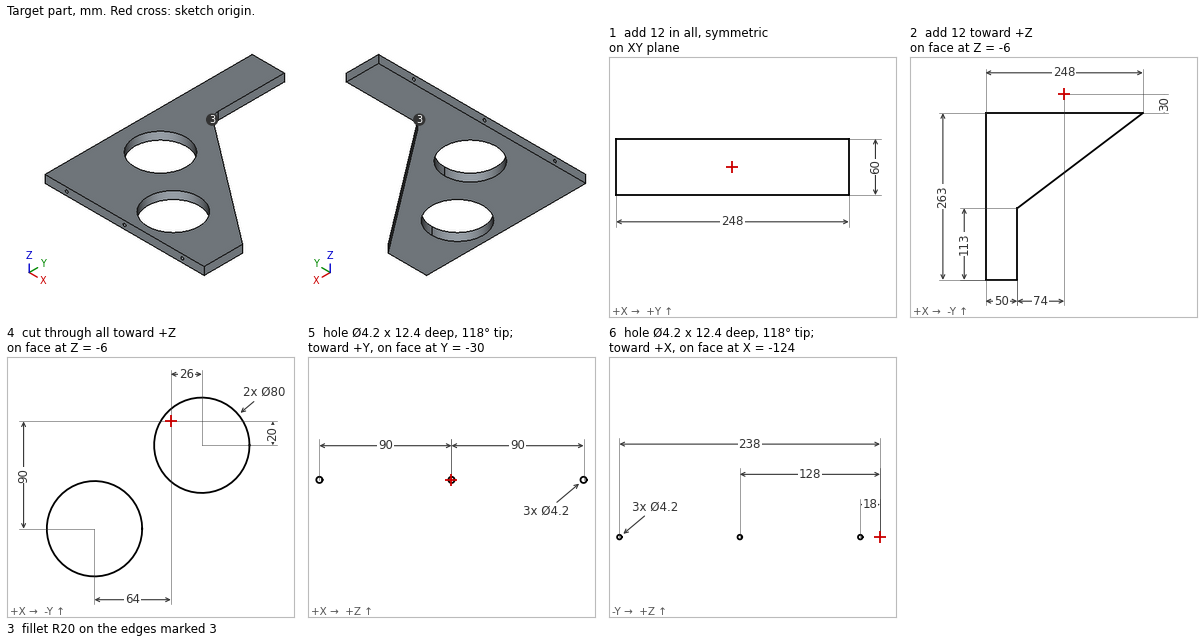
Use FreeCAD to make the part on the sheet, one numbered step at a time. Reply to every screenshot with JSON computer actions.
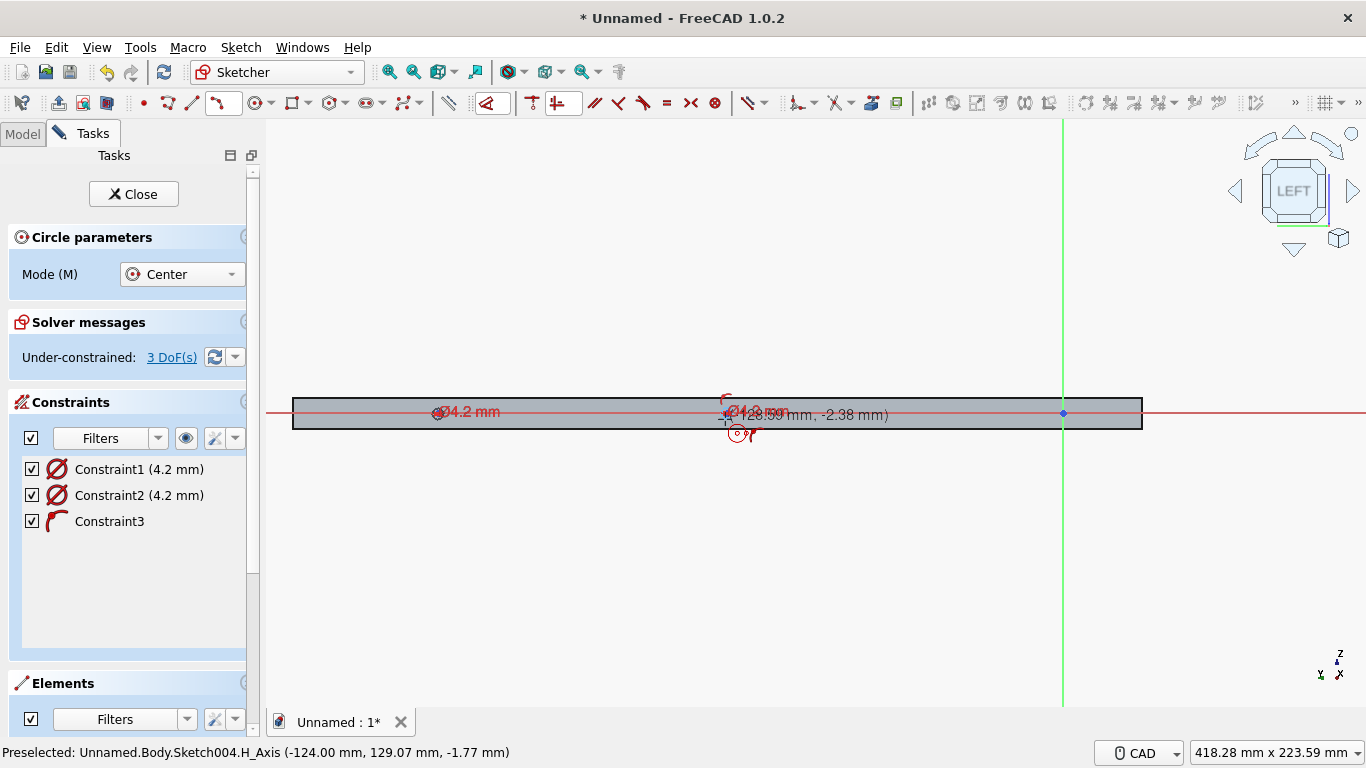
{"action": "scroll", "coordinate": [1016, 413], "scroll_direction": "up", "scroll_amount": 8}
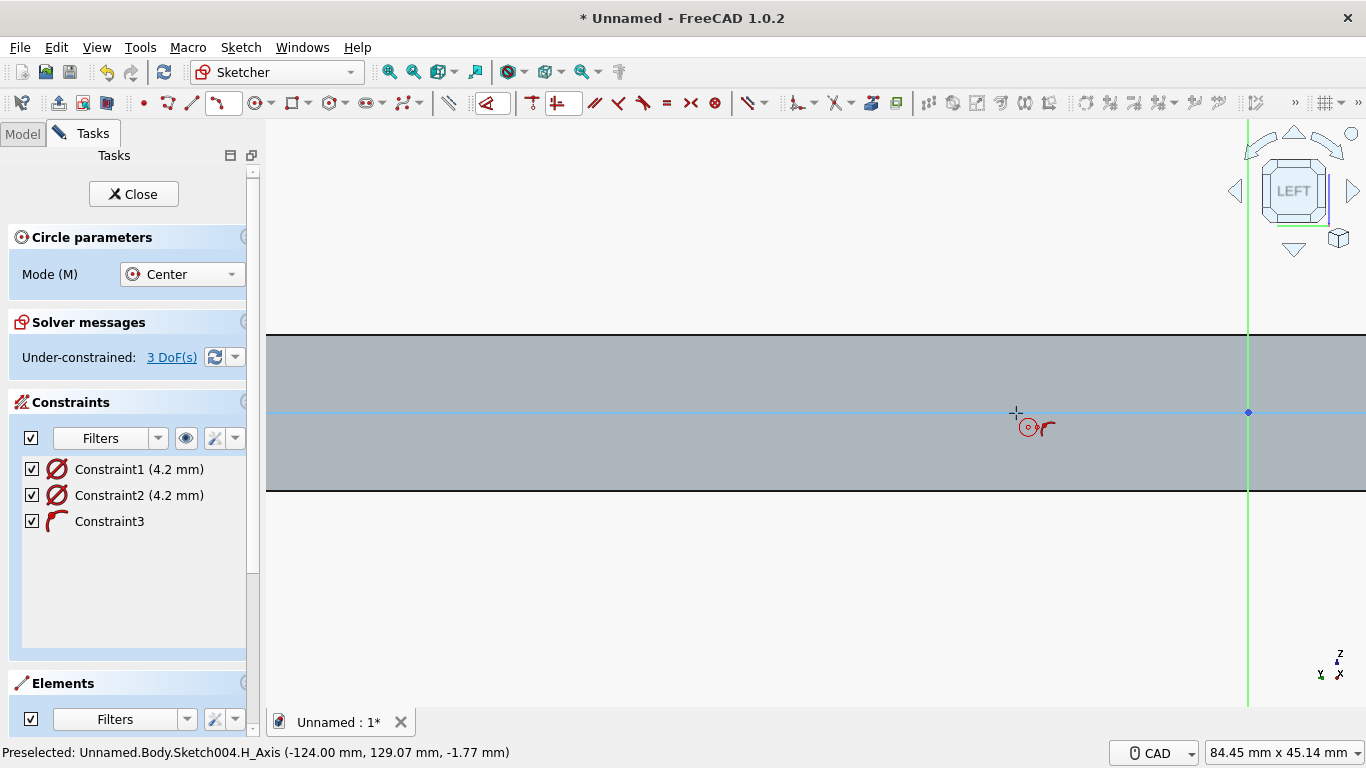
{"action": "scroll", "coordinate": [1016, 413], "scroll_direction": "down", "scroll_amount": 8}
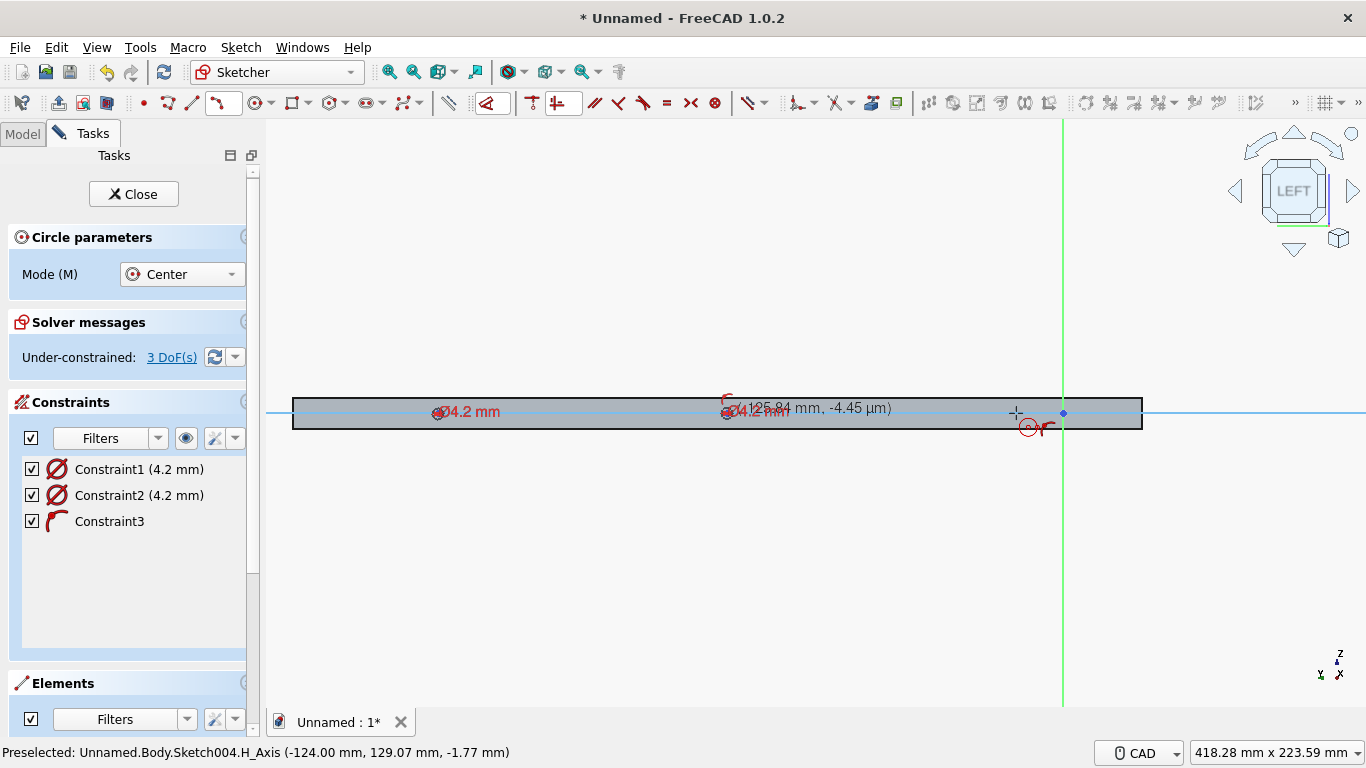
{"action": "left_click", "coordinate": [1016, 413]}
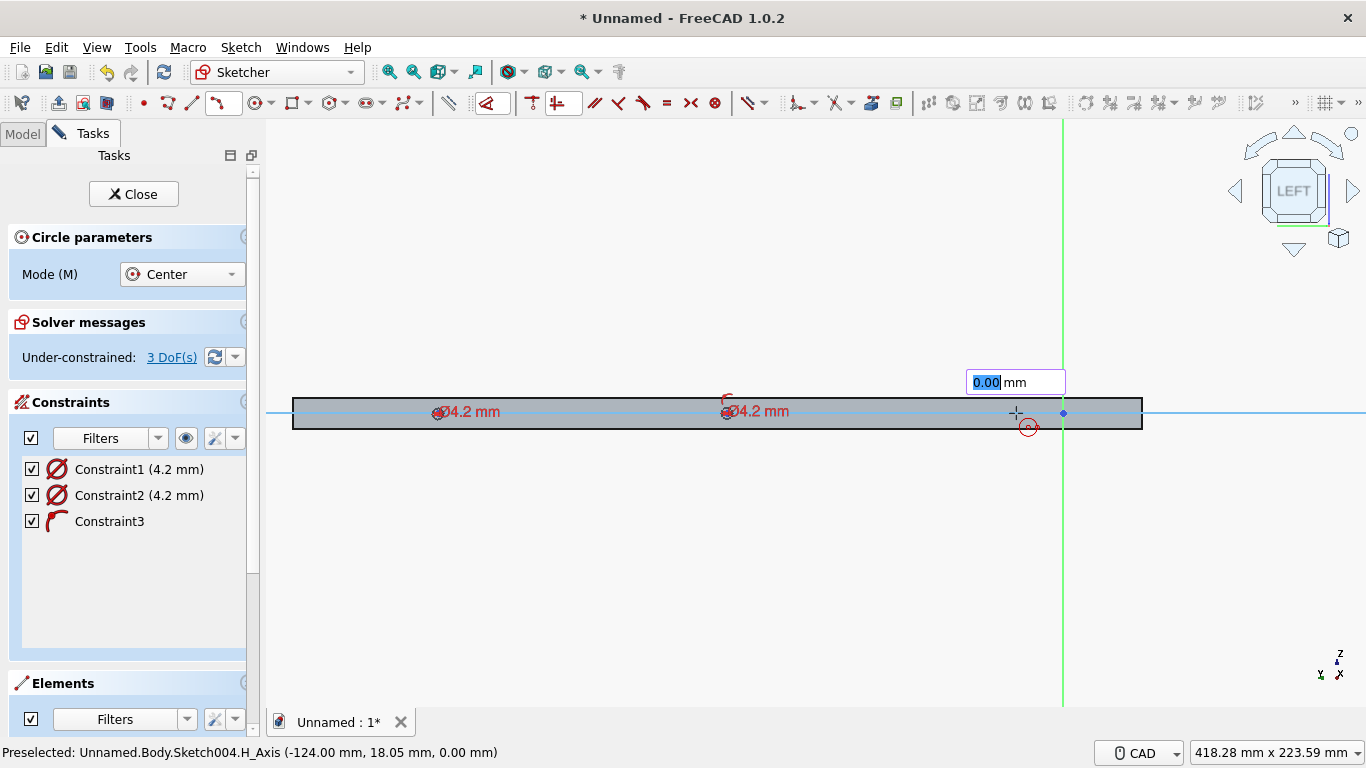
{"action": "scroll", "coordinate": [1014, 419], "scroll_direction": "up", "scroll_amount": 6}
{"action": "mouse_move", "coordinate": [1013, 416]}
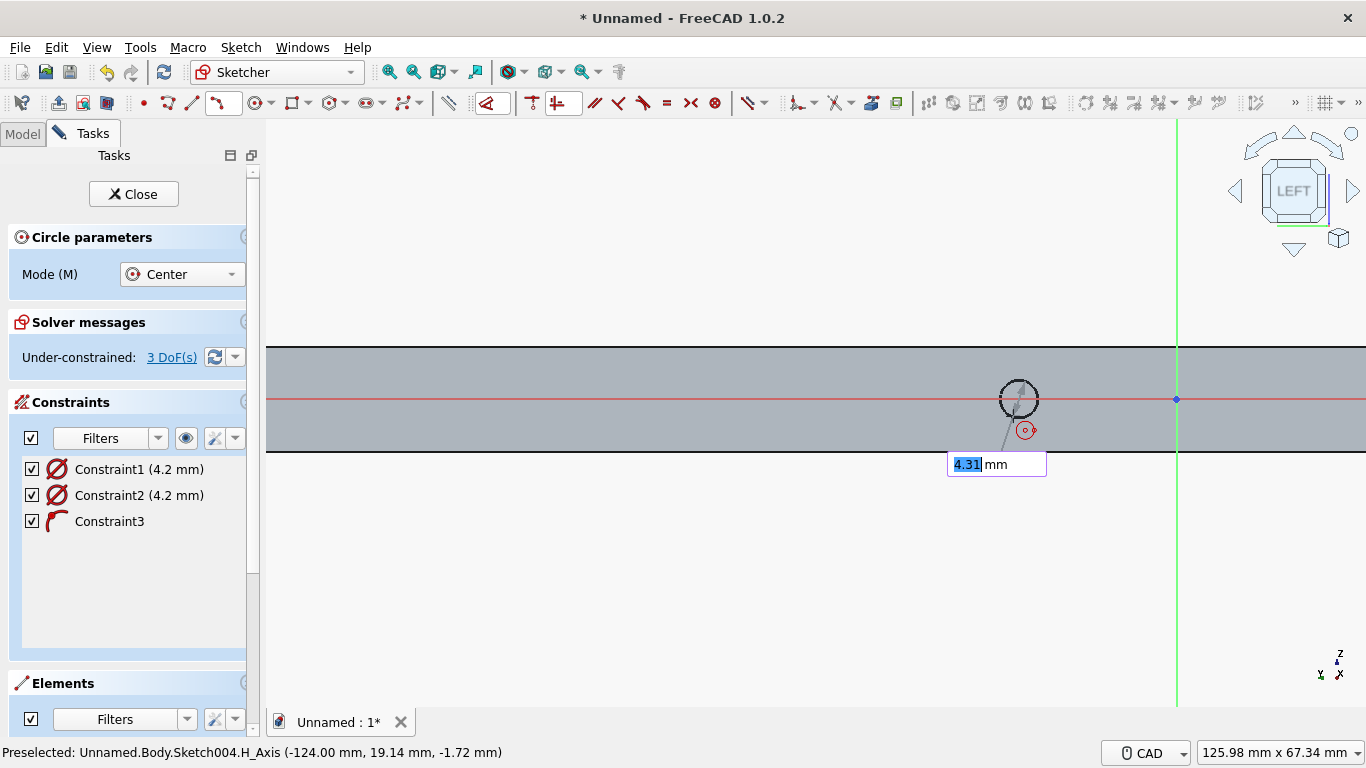
{"action": "type", "text": "4.2"}
{"action": "key", "text": "Return"}
{"action": "key", "text": "Escape"}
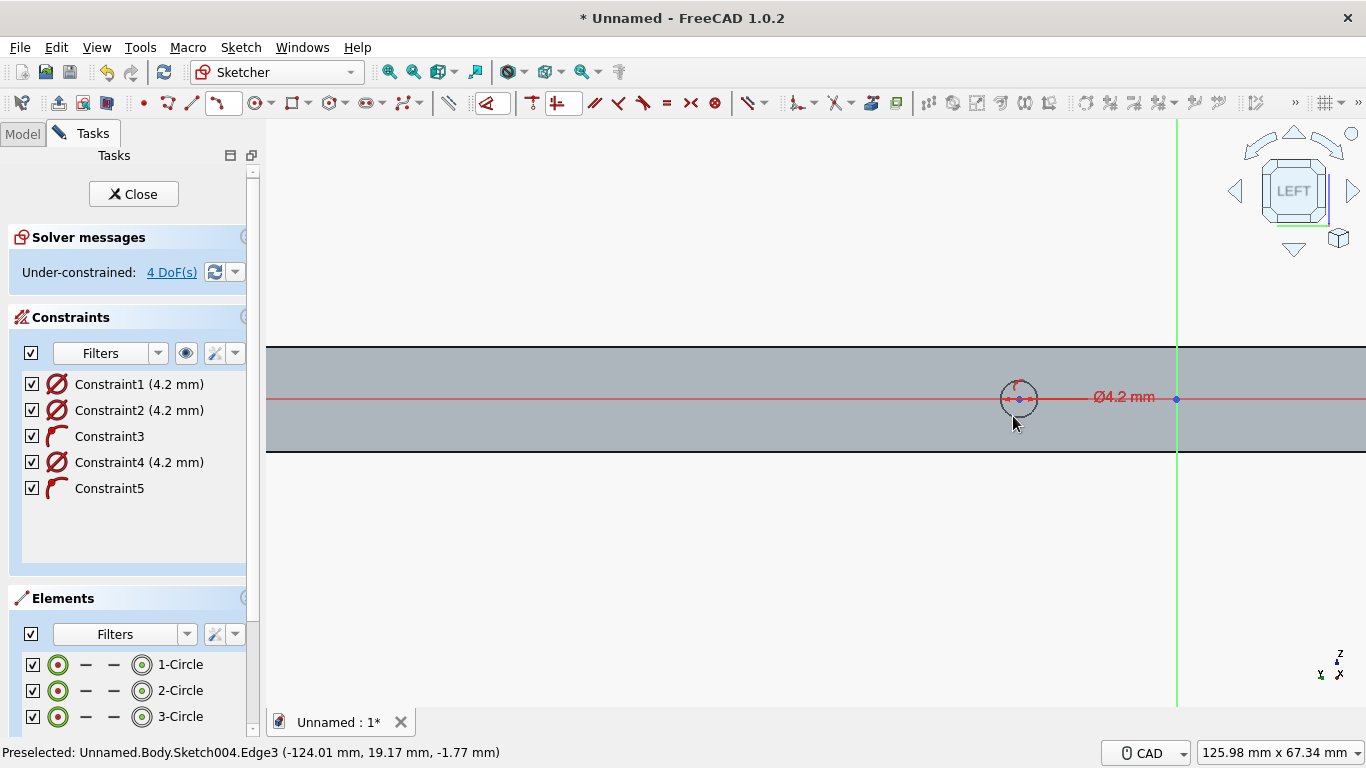
{"action": "scroll", "coordinate": [1014, 419], "scroll_direction": "down", "scroll_amount": 6}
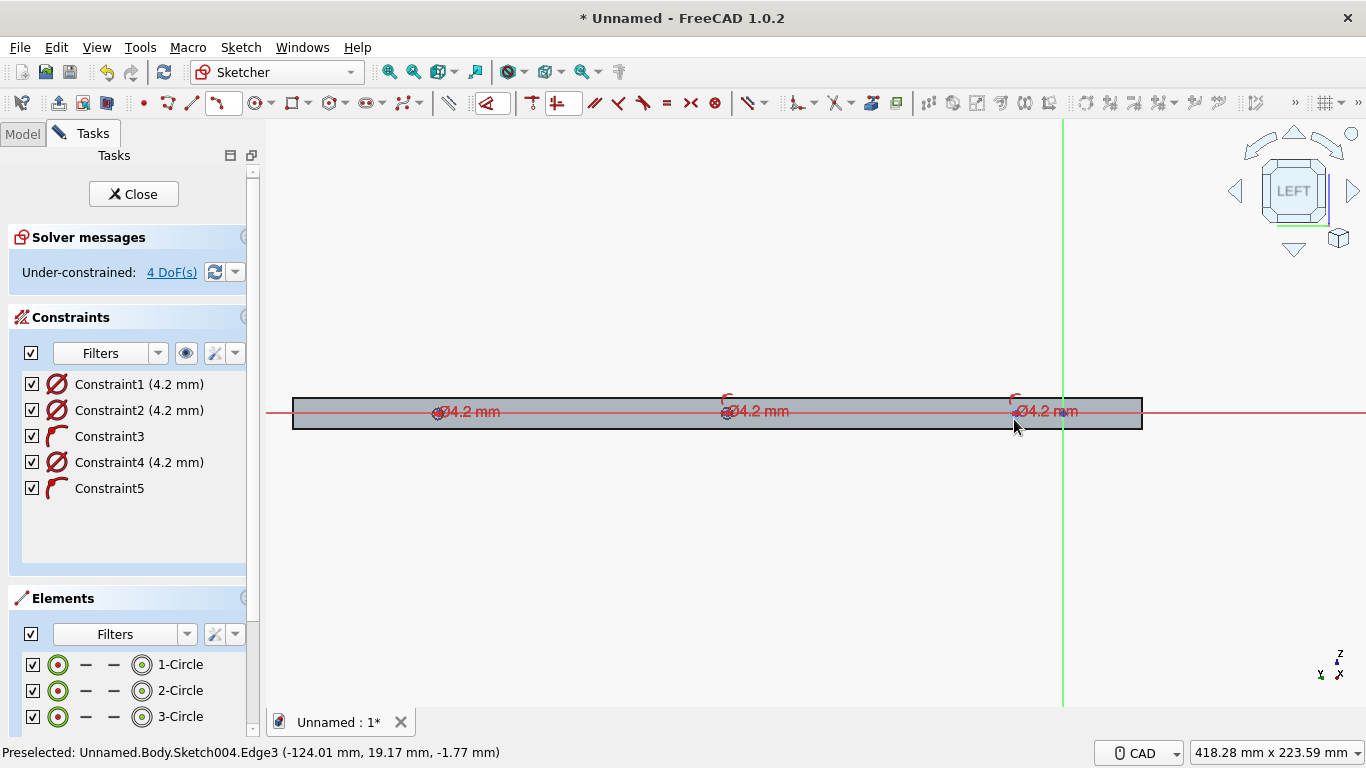
{"action": "left_click", "coordinate": [438, 414]}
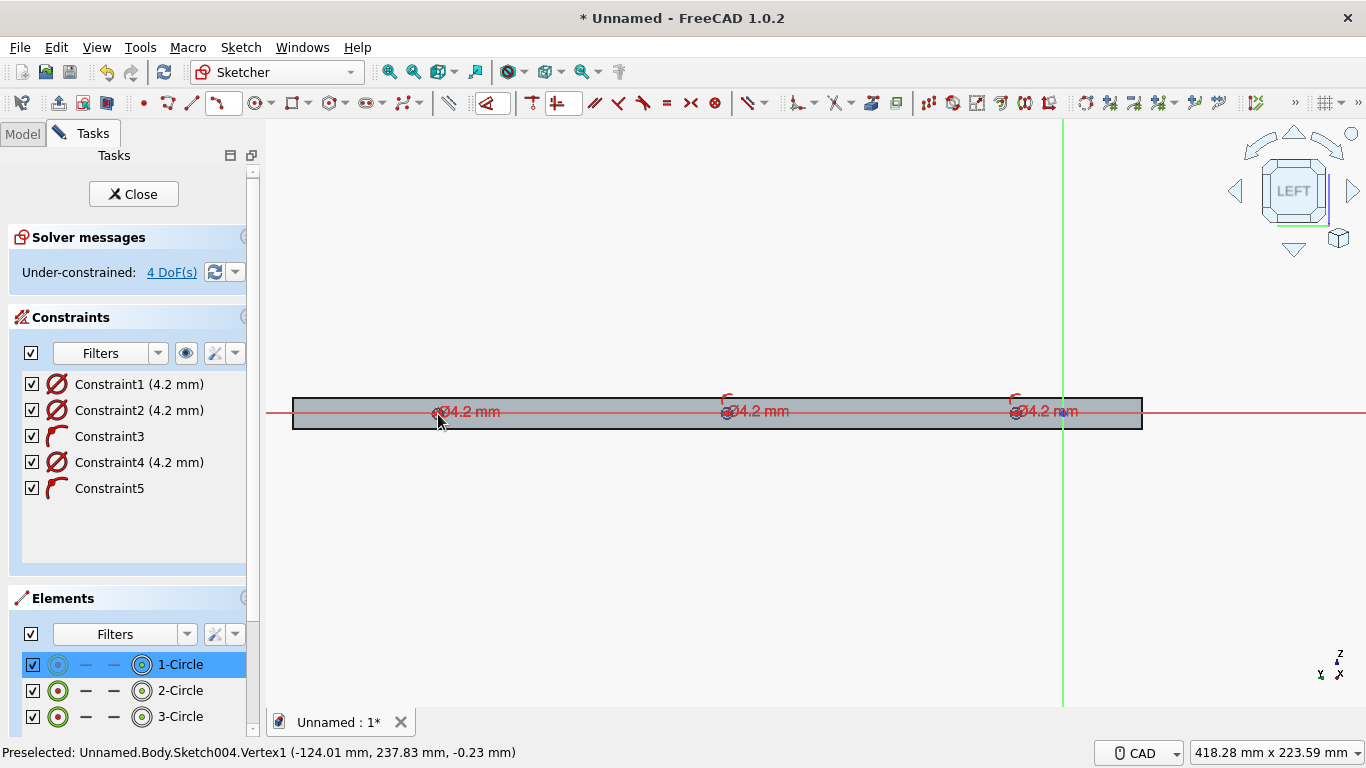
{"action": "left_click", "coordinate": [359, 413]}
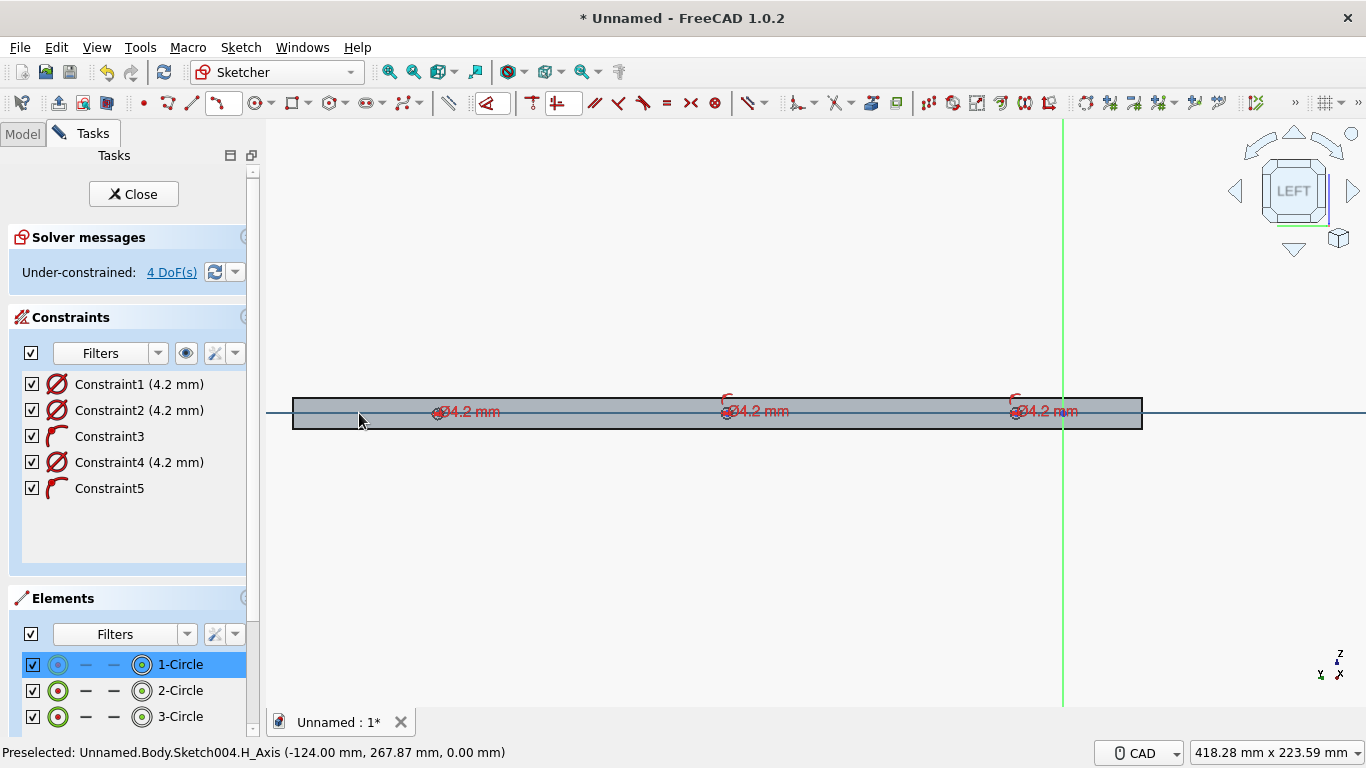
{"action": "key", "text": "c"}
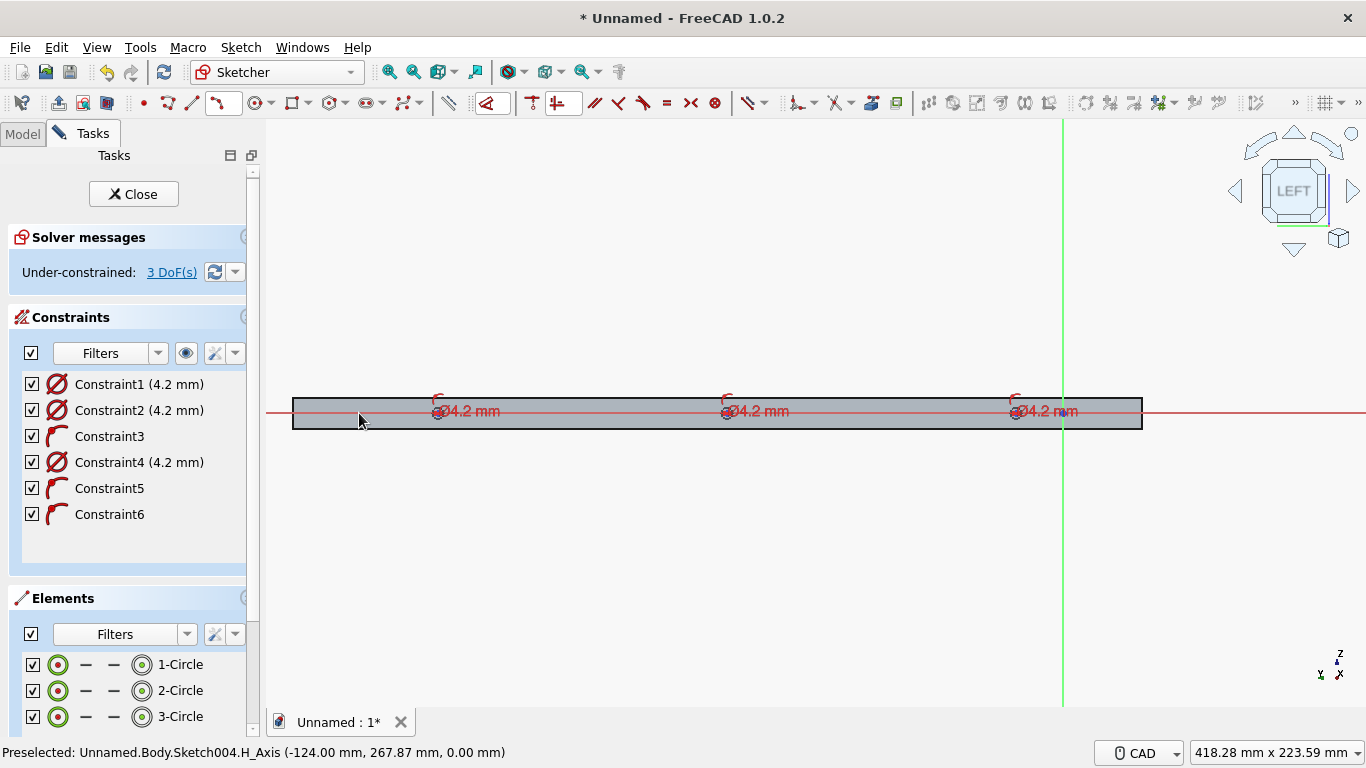
{"action": "left_click", "coordinate": [1016, 413]}